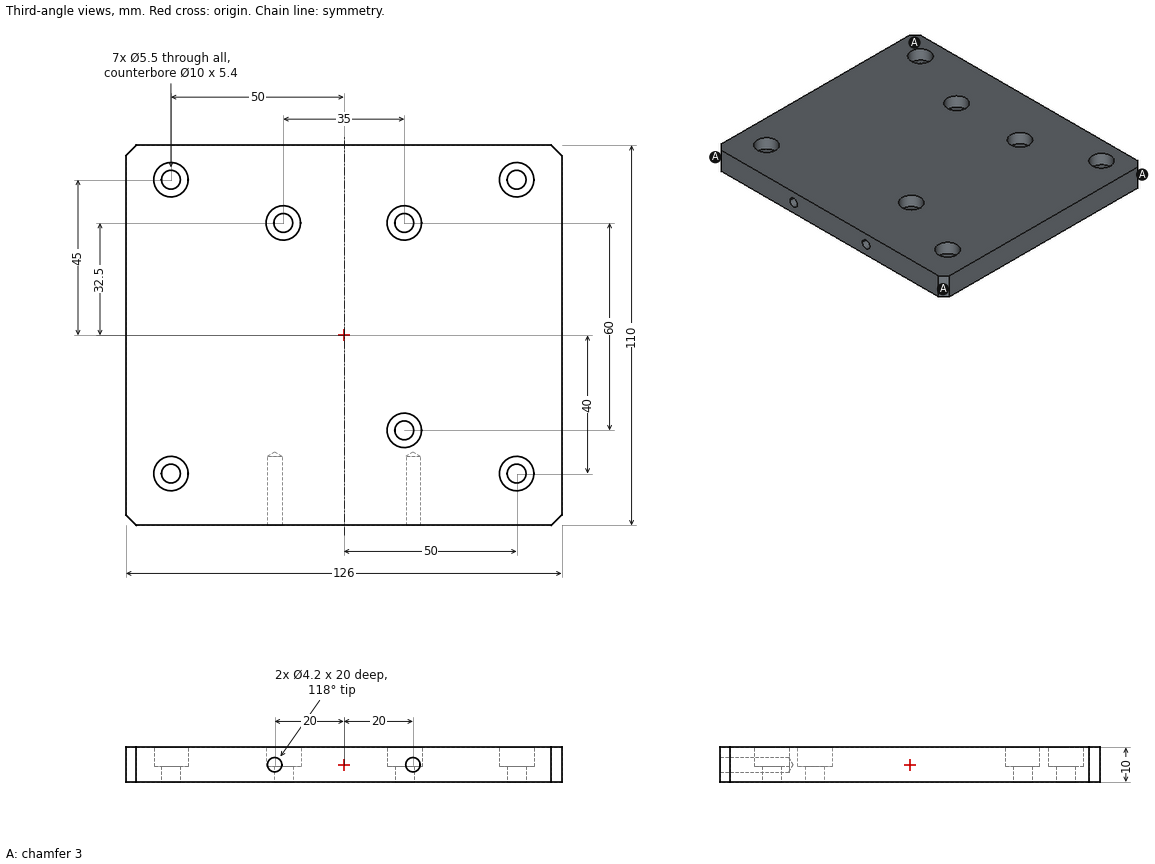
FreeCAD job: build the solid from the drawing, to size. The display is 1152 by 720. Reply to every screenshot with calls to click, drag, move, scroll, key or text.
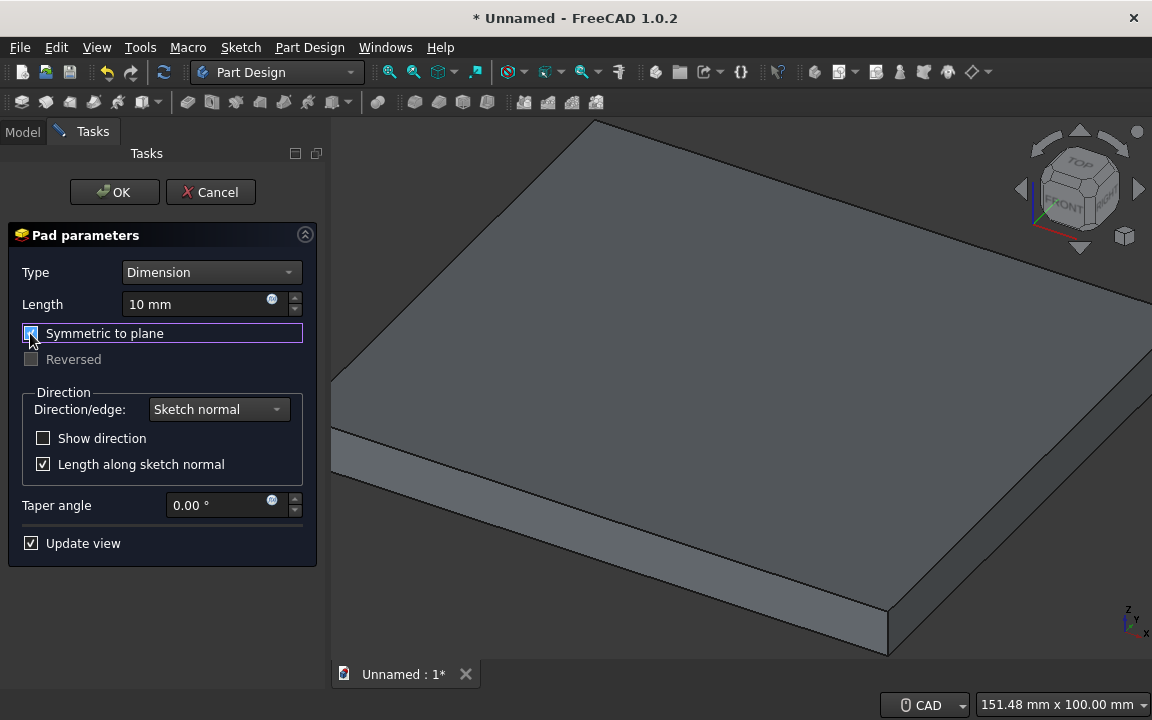
click(115, 192)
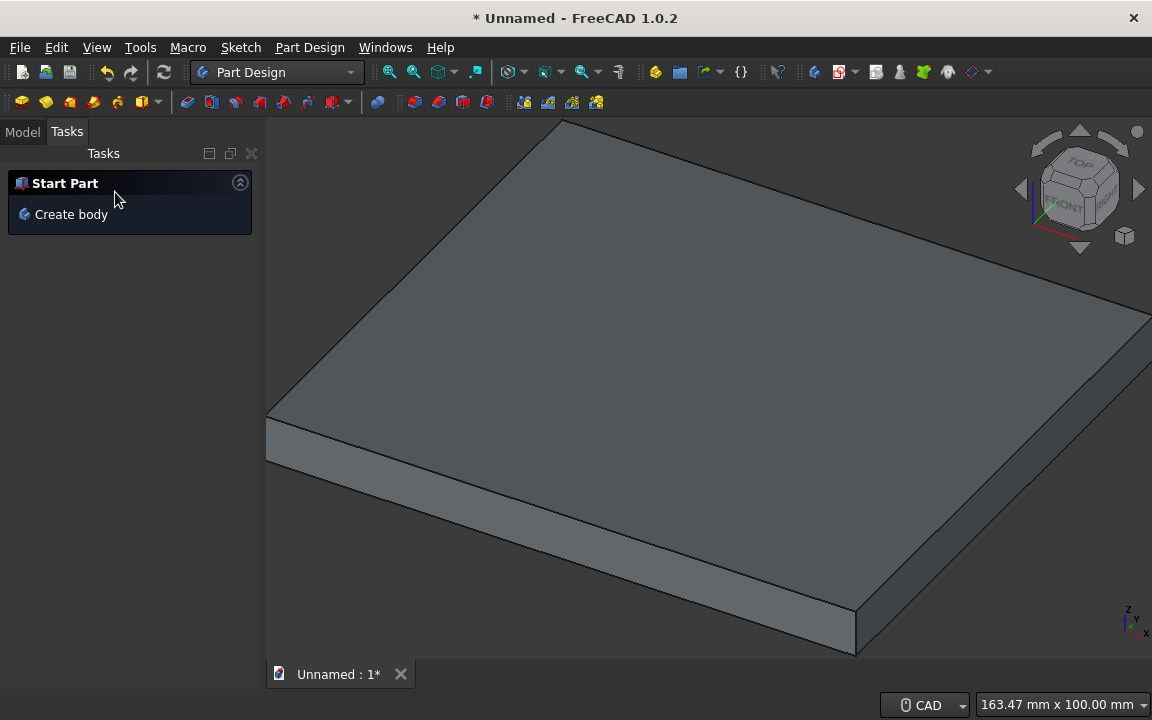
click(390, 72)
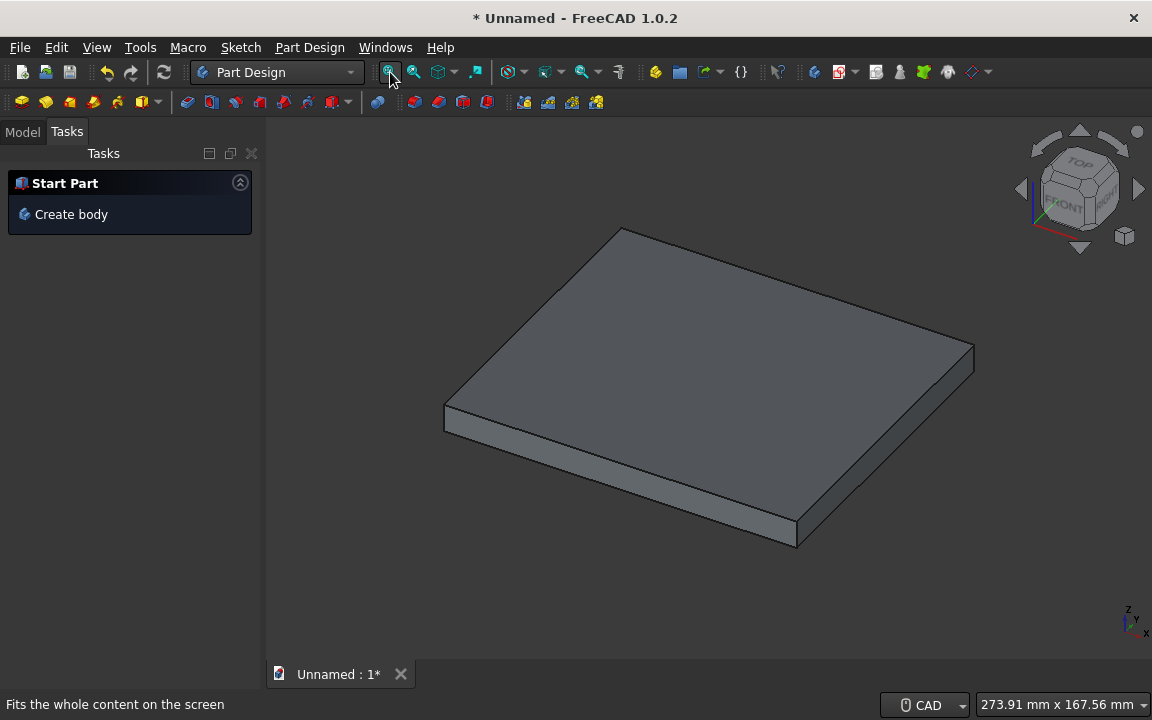
click(797, 534)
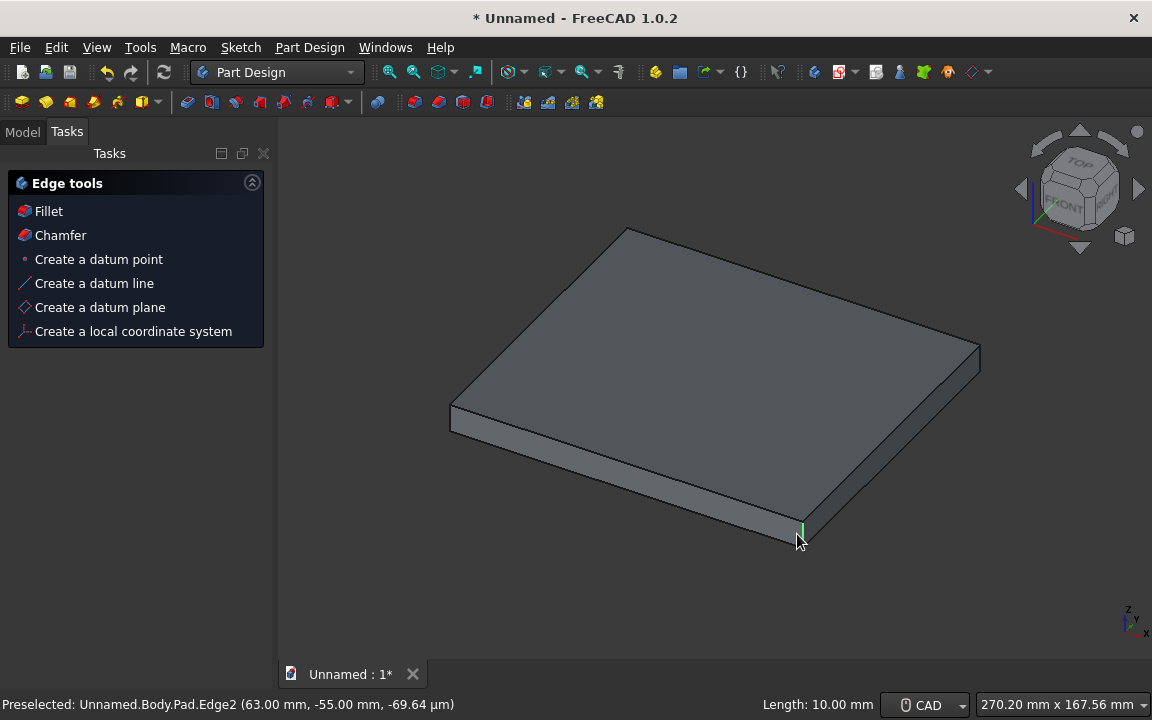
key(0)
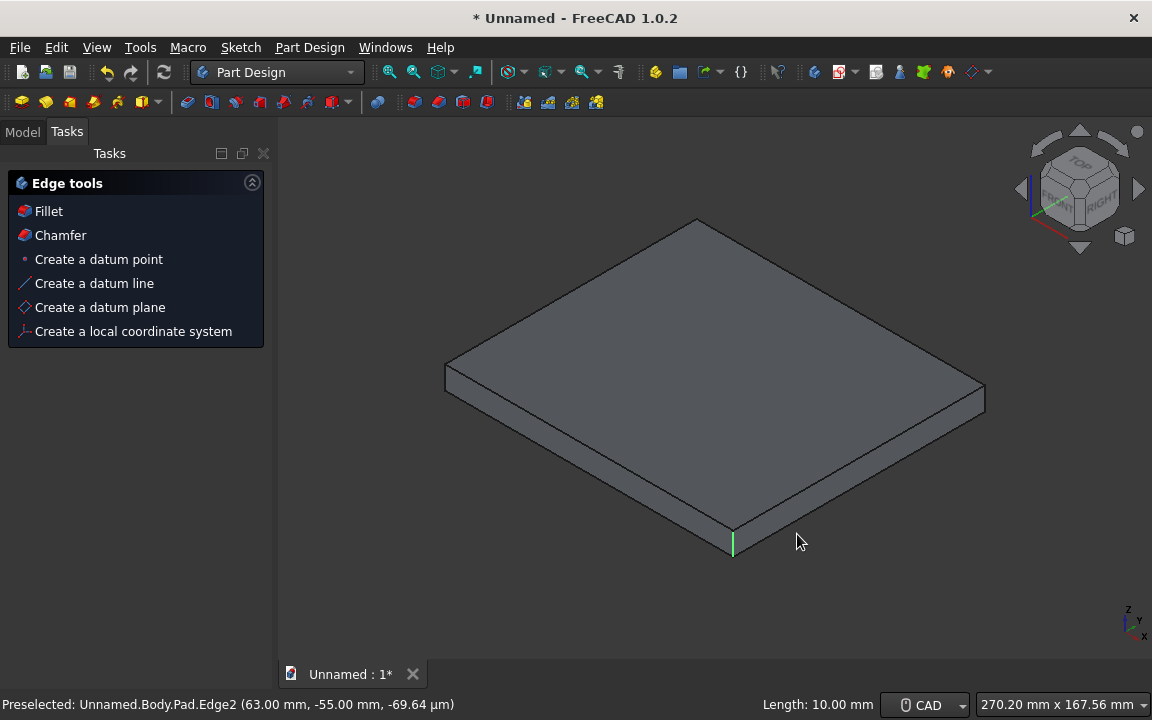
key(2)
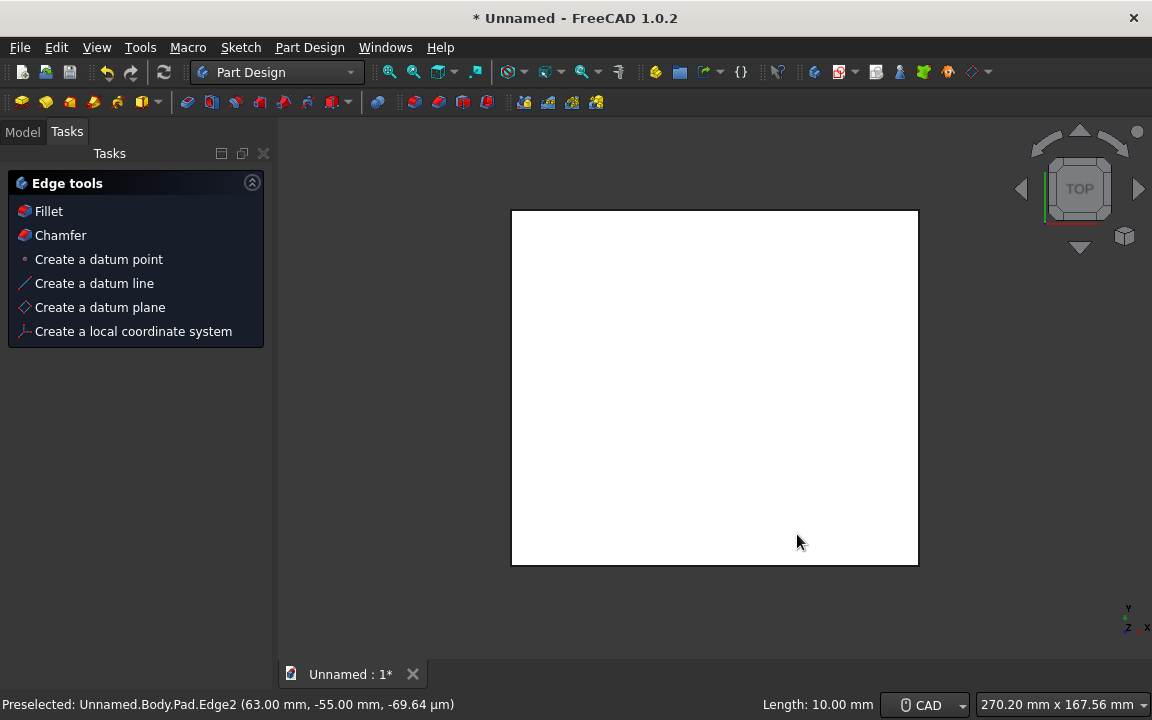
key(1)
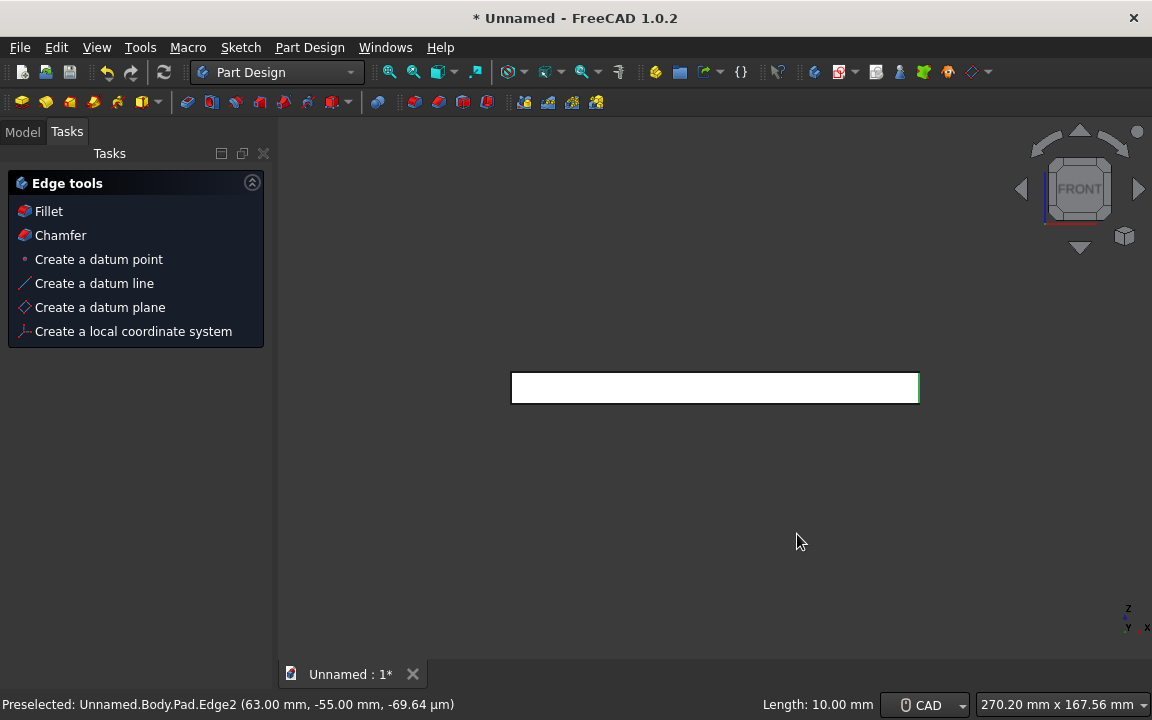
click(511, 387, ctrl)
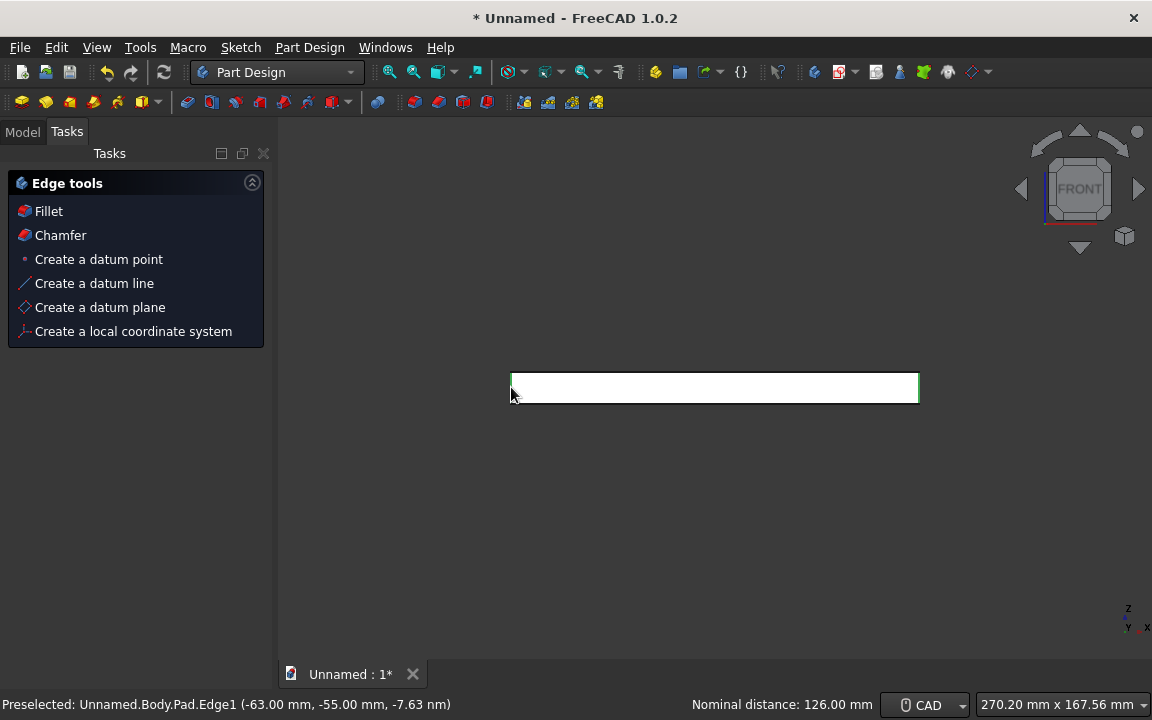
key(3)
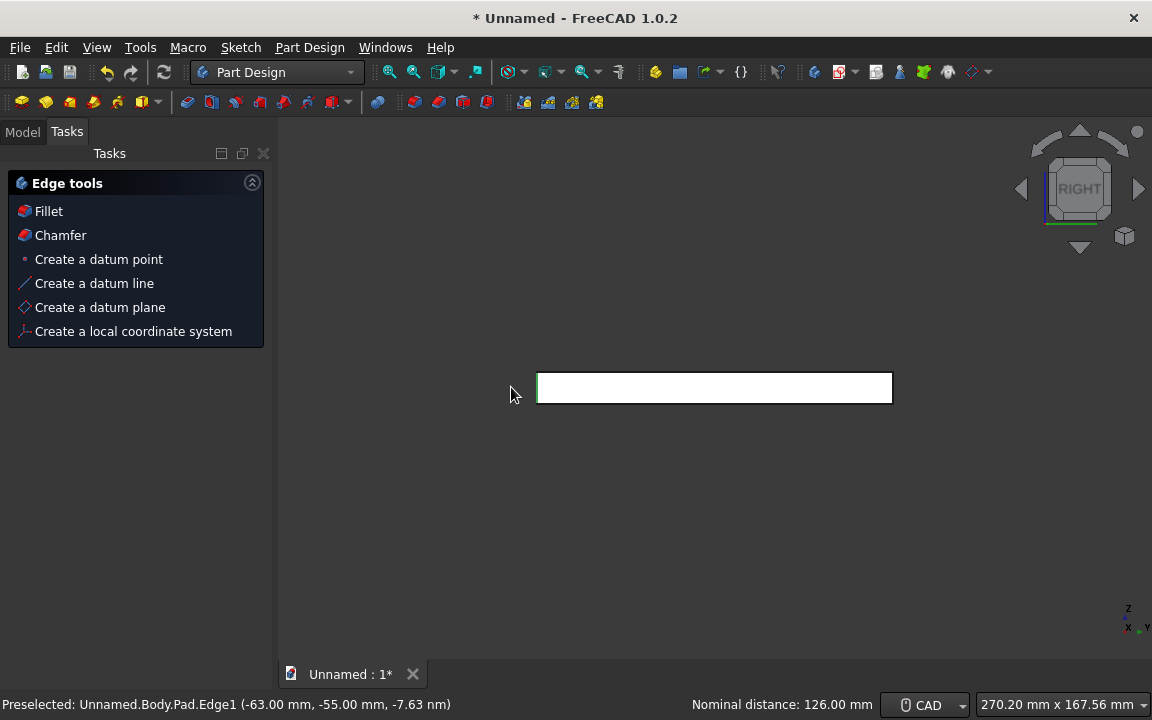
click(390, 72)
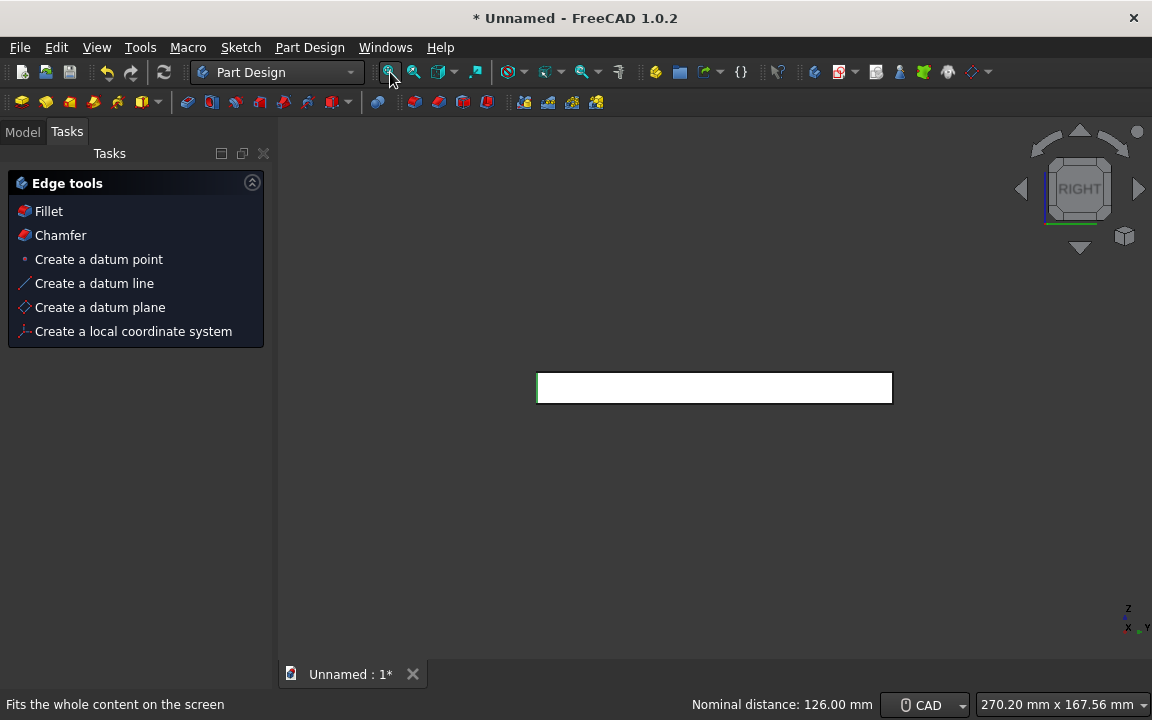
click(893, 387, ctrl)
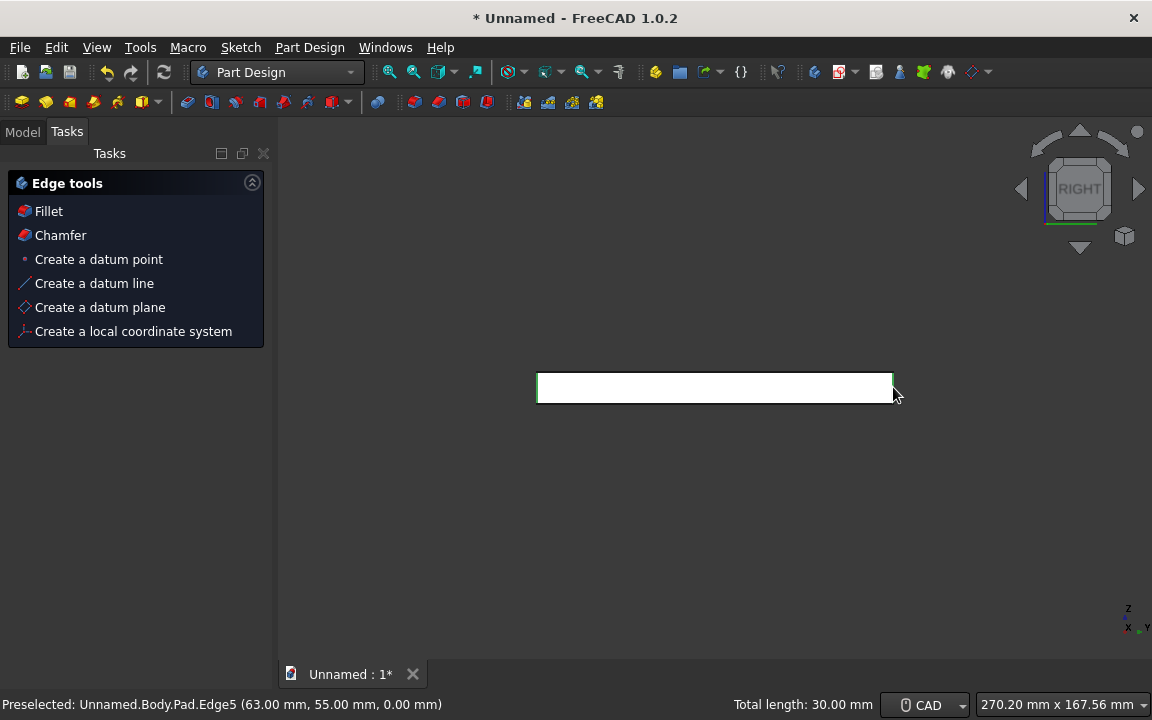
key(5)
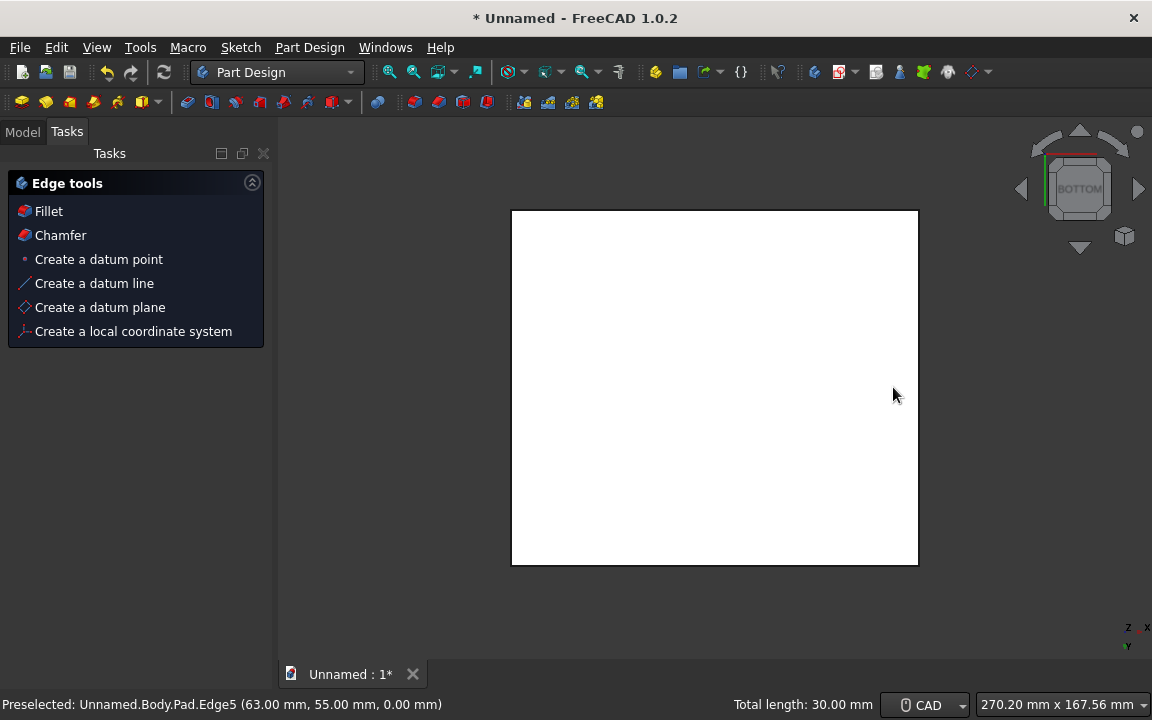
key(4)